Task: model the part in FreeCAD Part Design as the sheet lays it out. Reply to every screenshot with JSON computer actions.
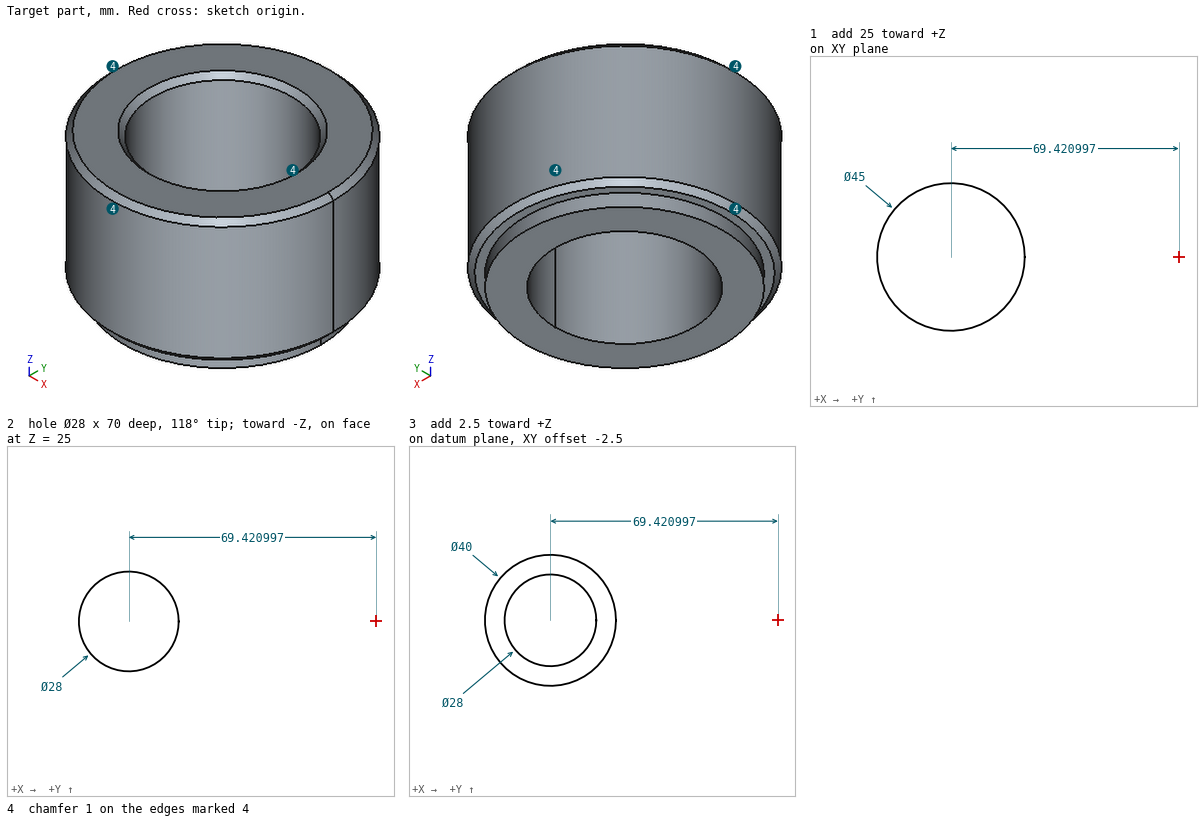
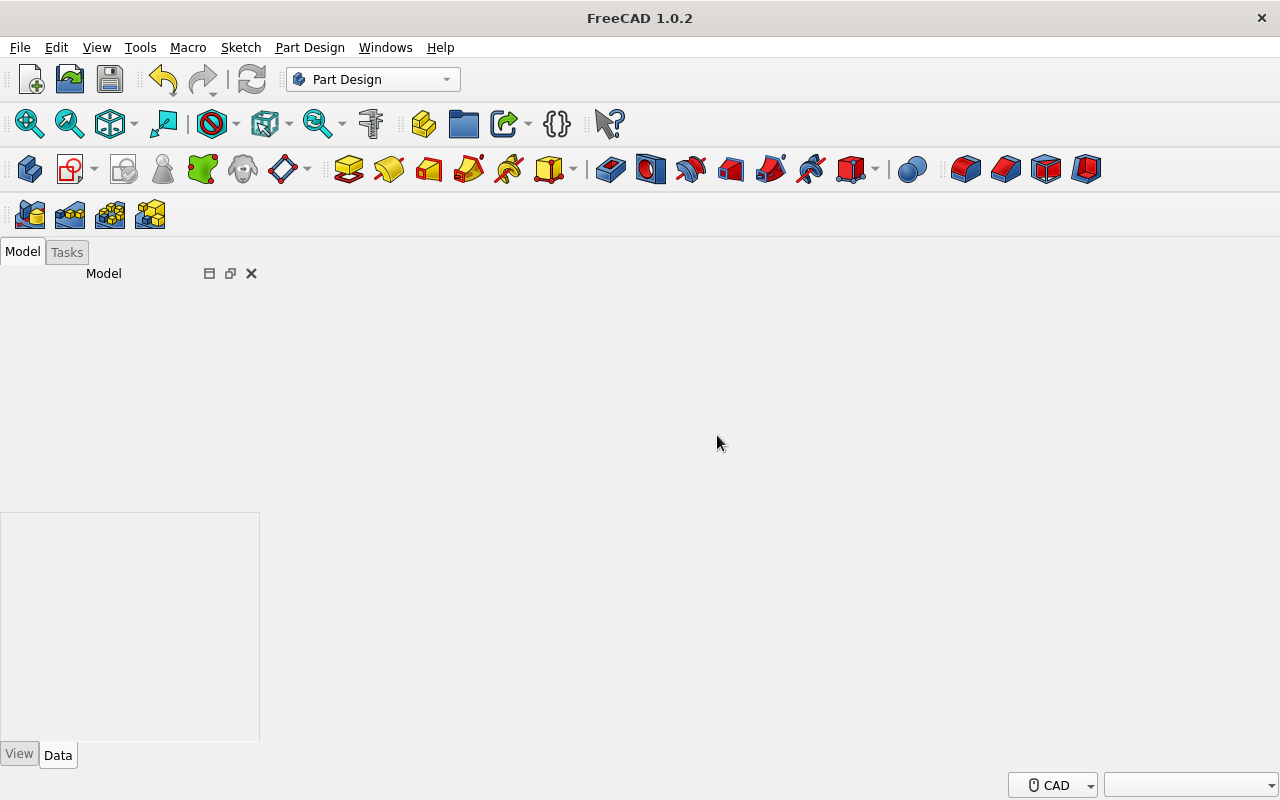
{"action": "key", "text": "ctrl+n"}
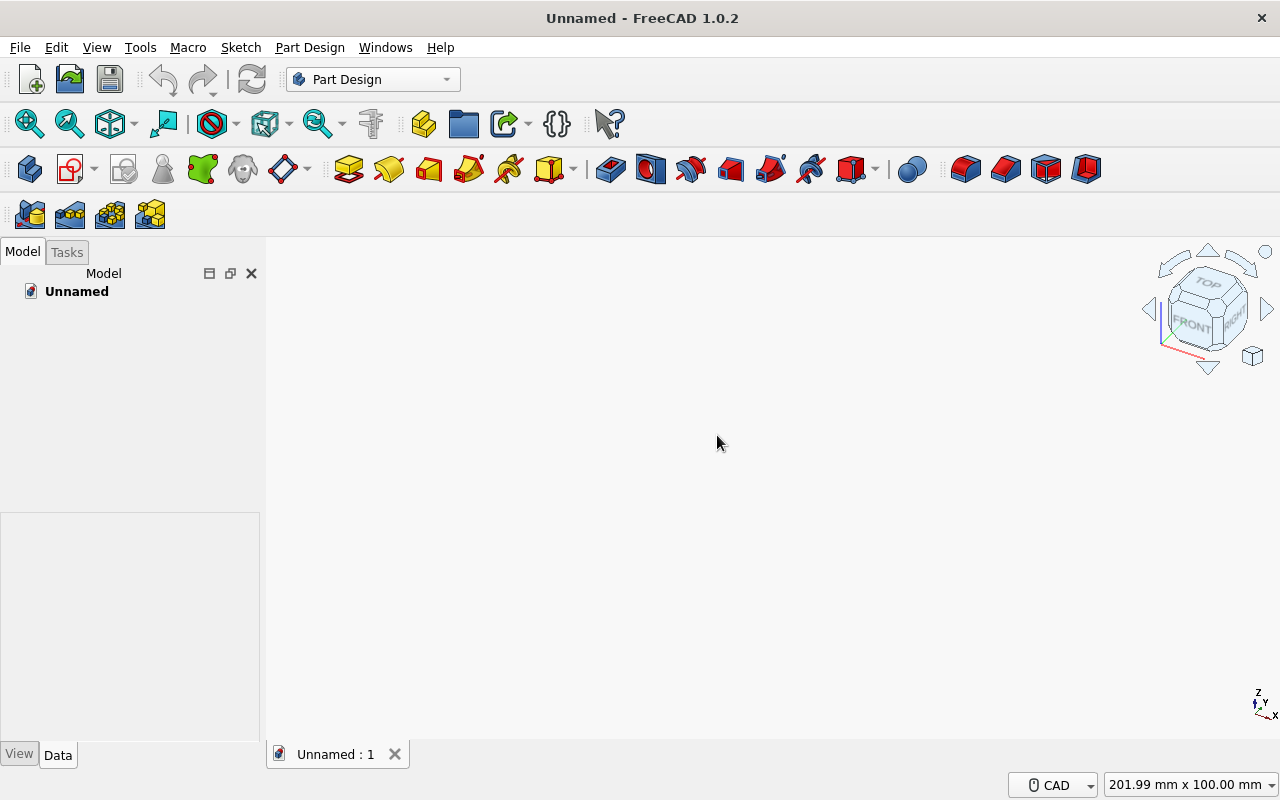
{"action": "left_click", "coordinate": [70, 170]}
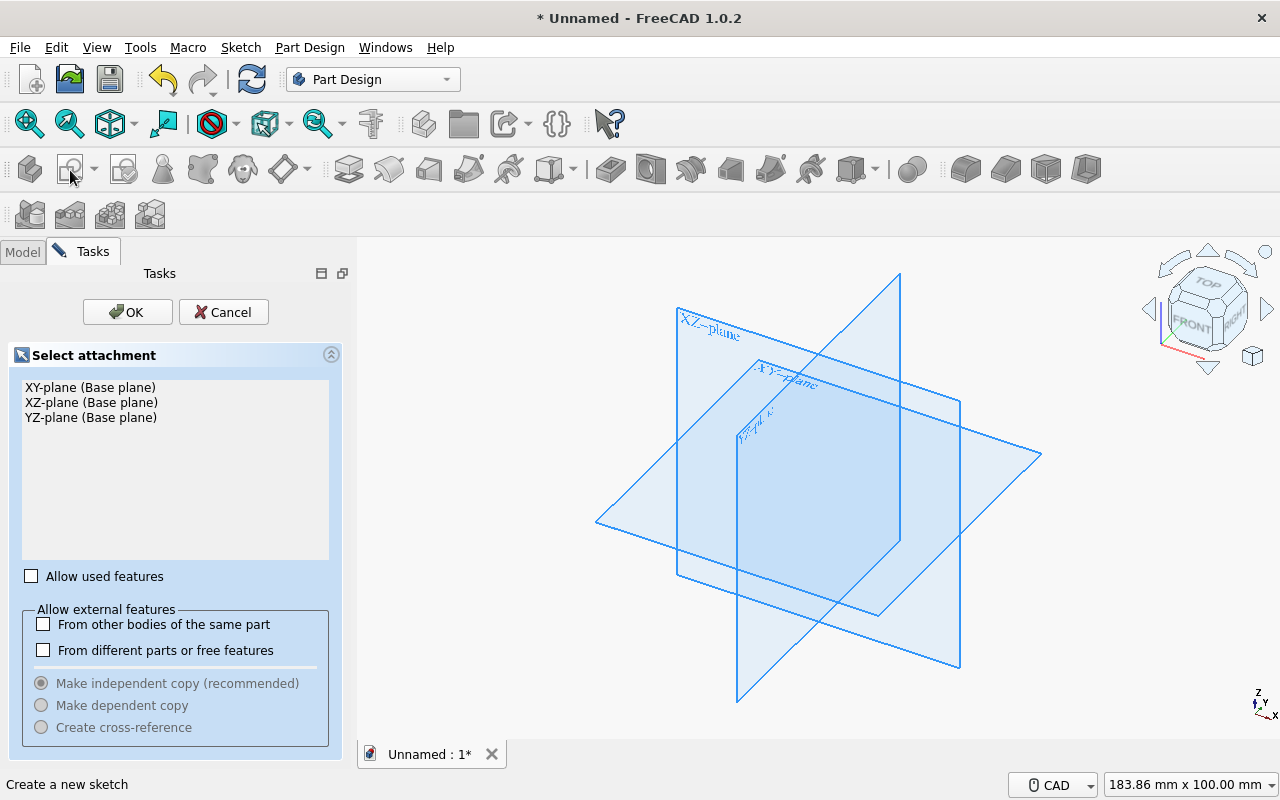
{"action": "left_click", "coordinate": [82, 388]}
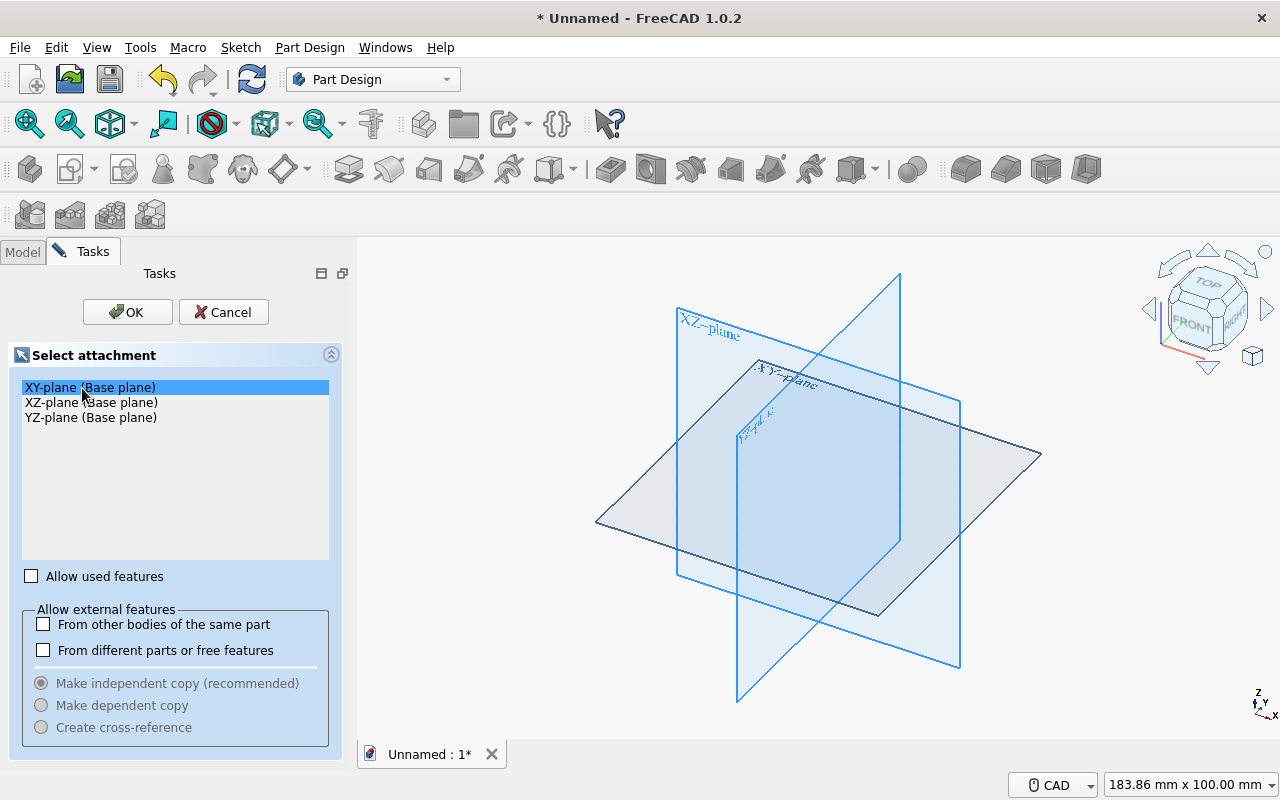
{"action": "left_click", "coordinate": [128, 312]}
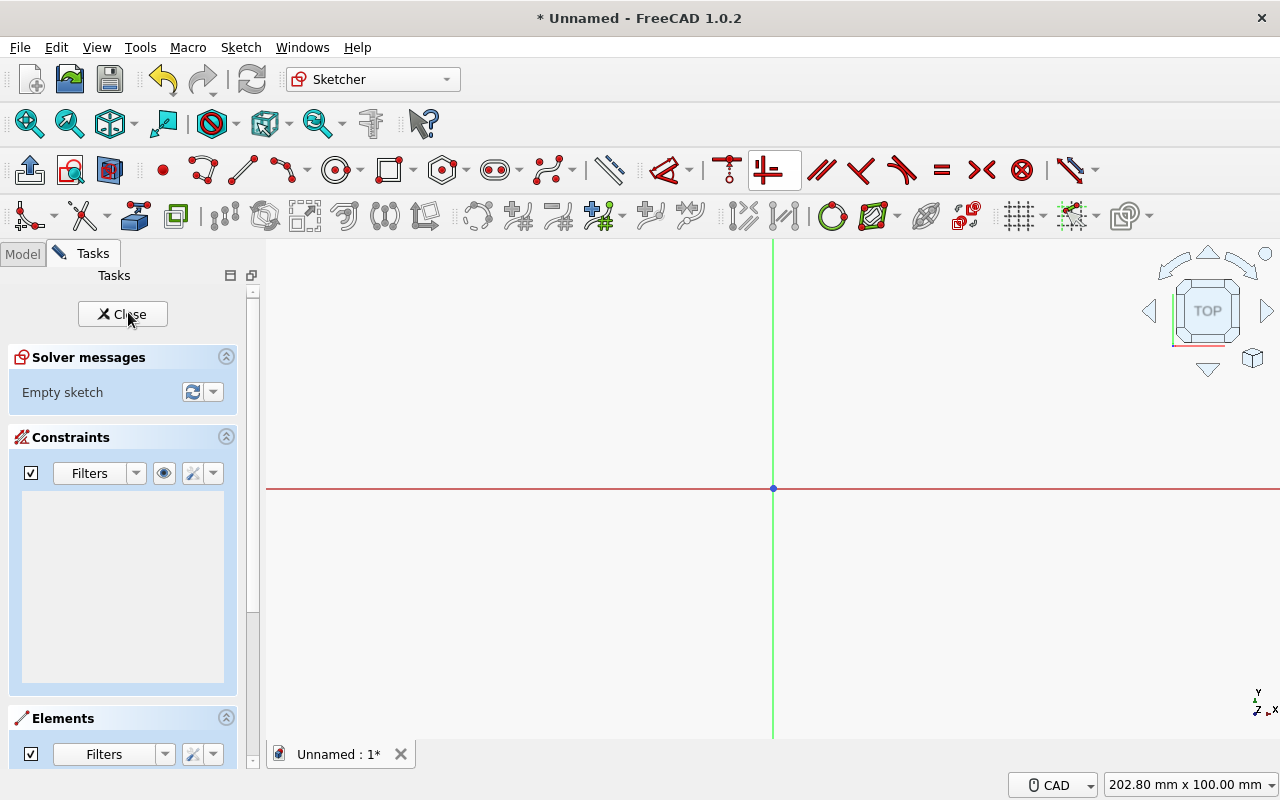
{"action": "scroll", "coordinate": [1115, 489], "scroll_direction": "down", "scroll_amount": 1}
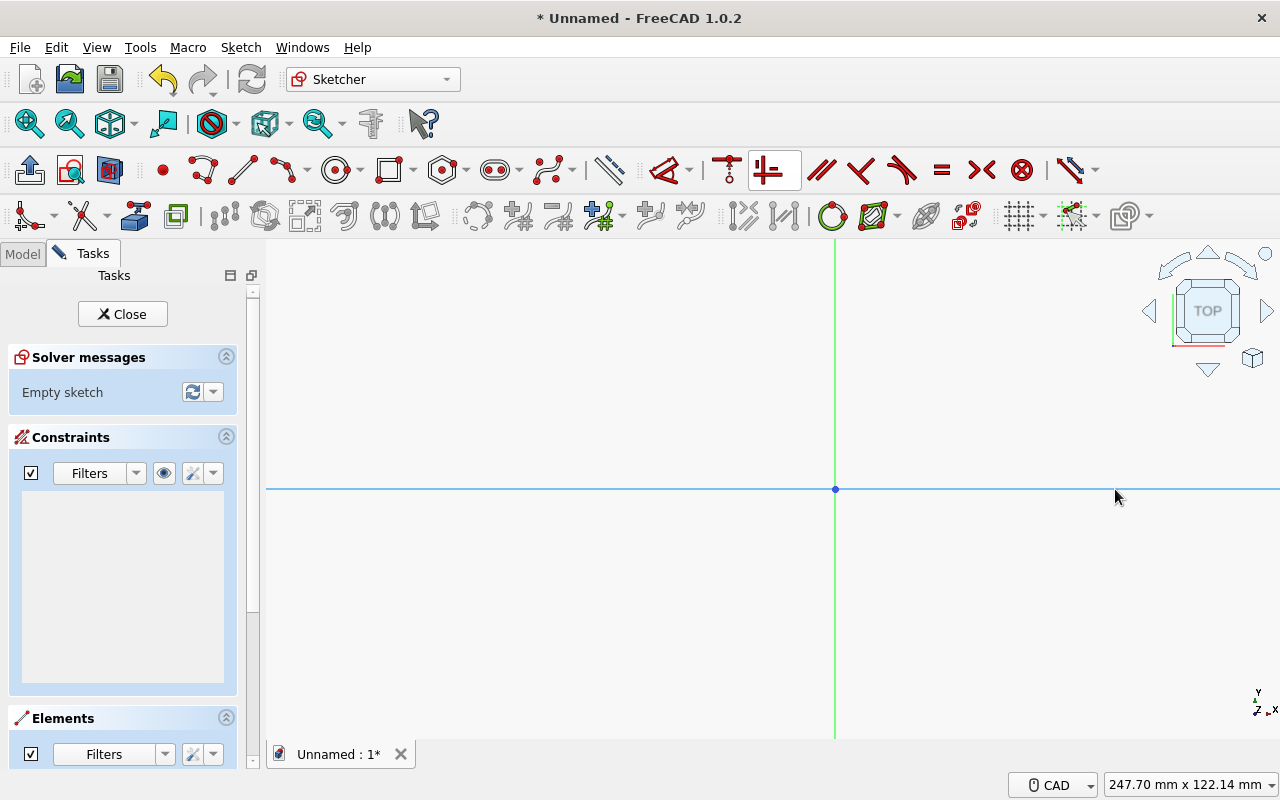
{"action": "scroll", "coordinate": [530, 489], "scroll_direction": "up", "scroll_amount": 2}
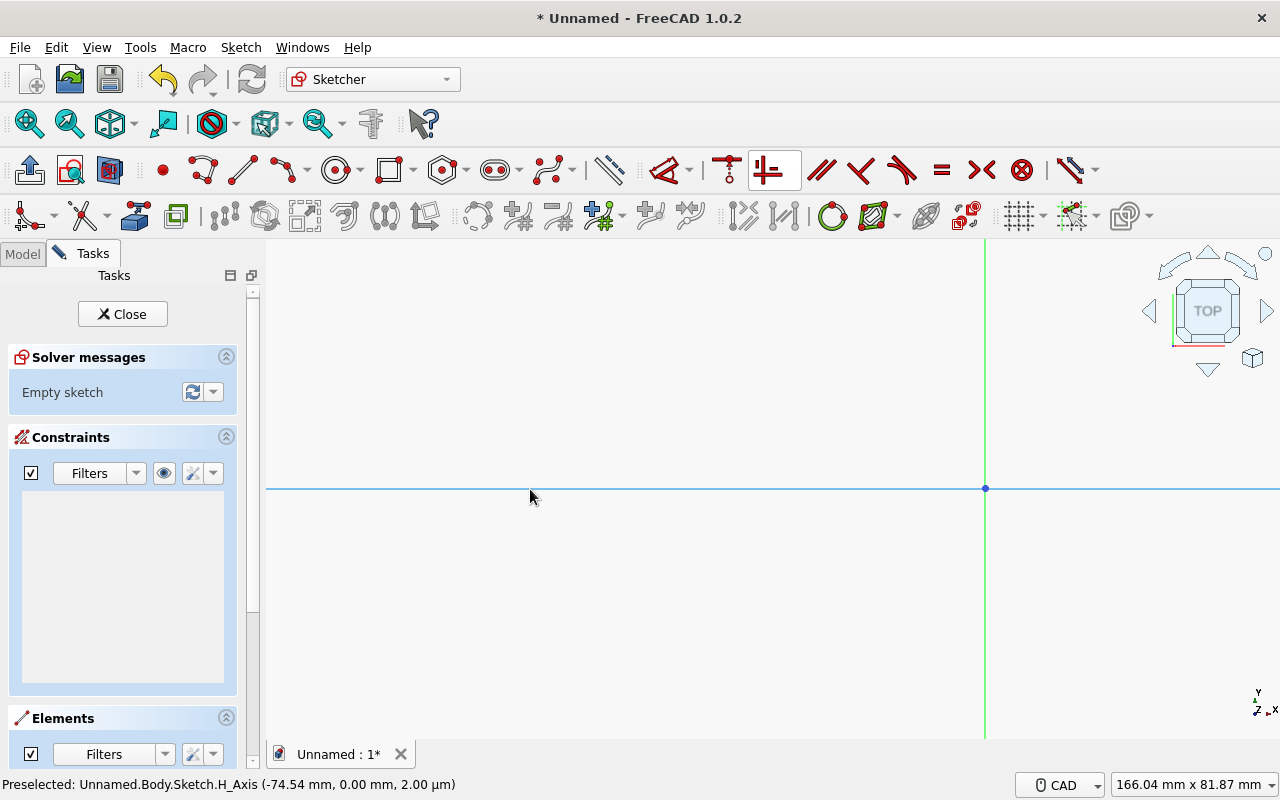
{"action": "key", "text": "g c"}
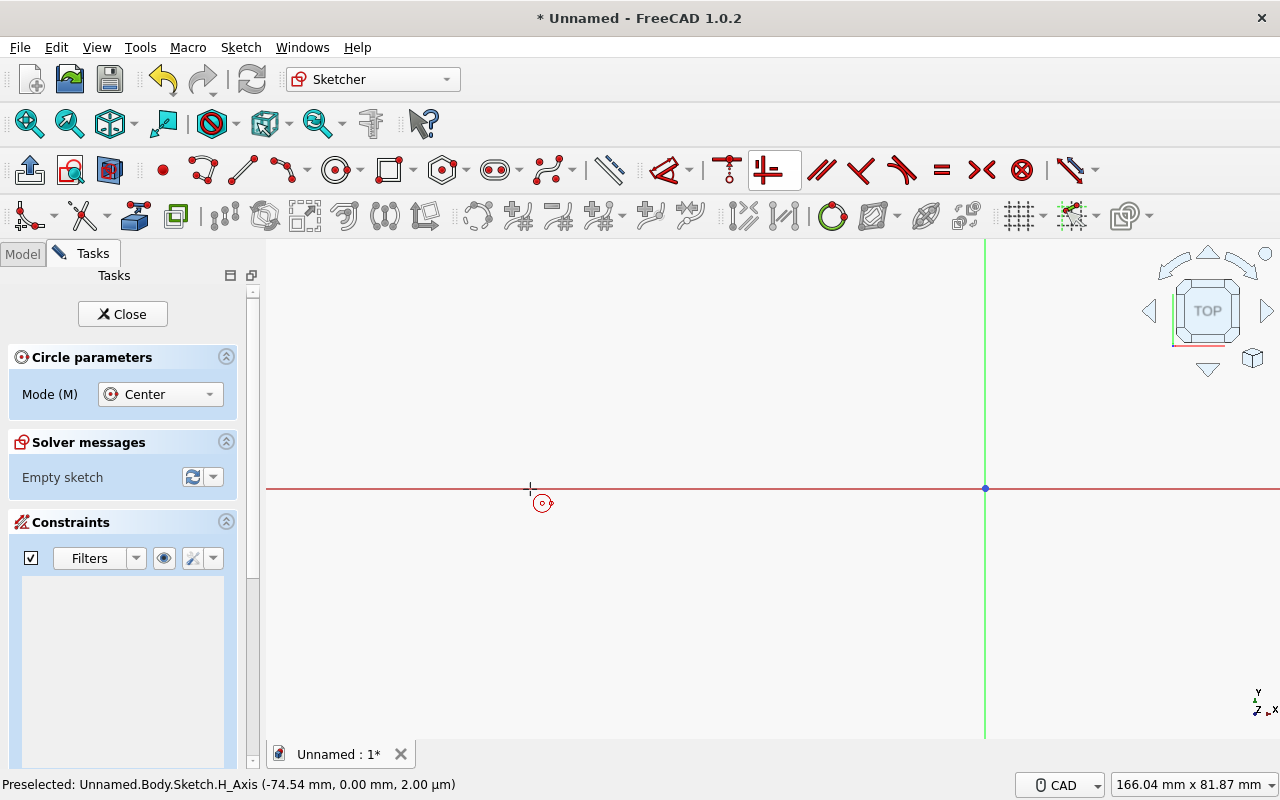
{"action": "left_click", "coordinate": [561, 489]}
{"action": "mouse_move", "coordinate": [658, 392]}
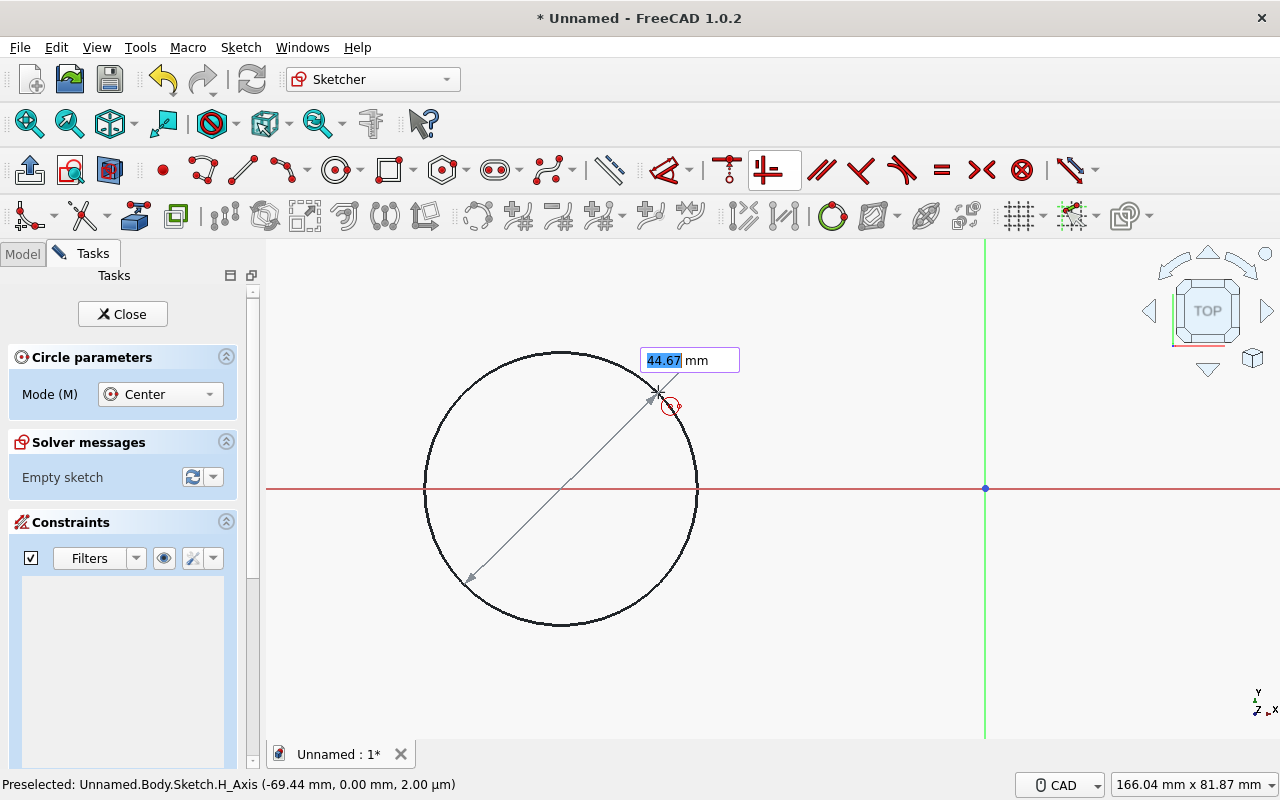
{"action": "type", "text": "45"}
{"action": "key", "text": "Return"}
{"action": "key", "text": "Escape"}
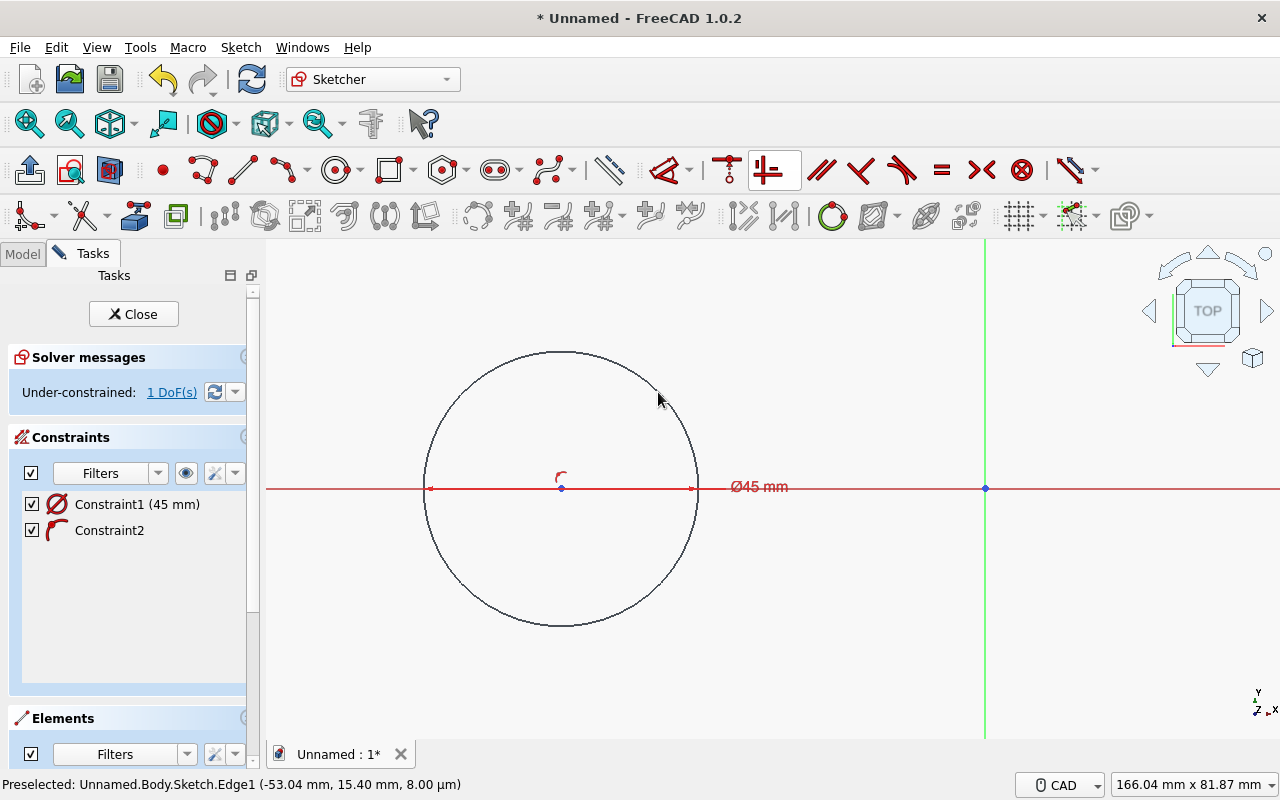
{"action": "left_click", "coordinate": [664, 170]}